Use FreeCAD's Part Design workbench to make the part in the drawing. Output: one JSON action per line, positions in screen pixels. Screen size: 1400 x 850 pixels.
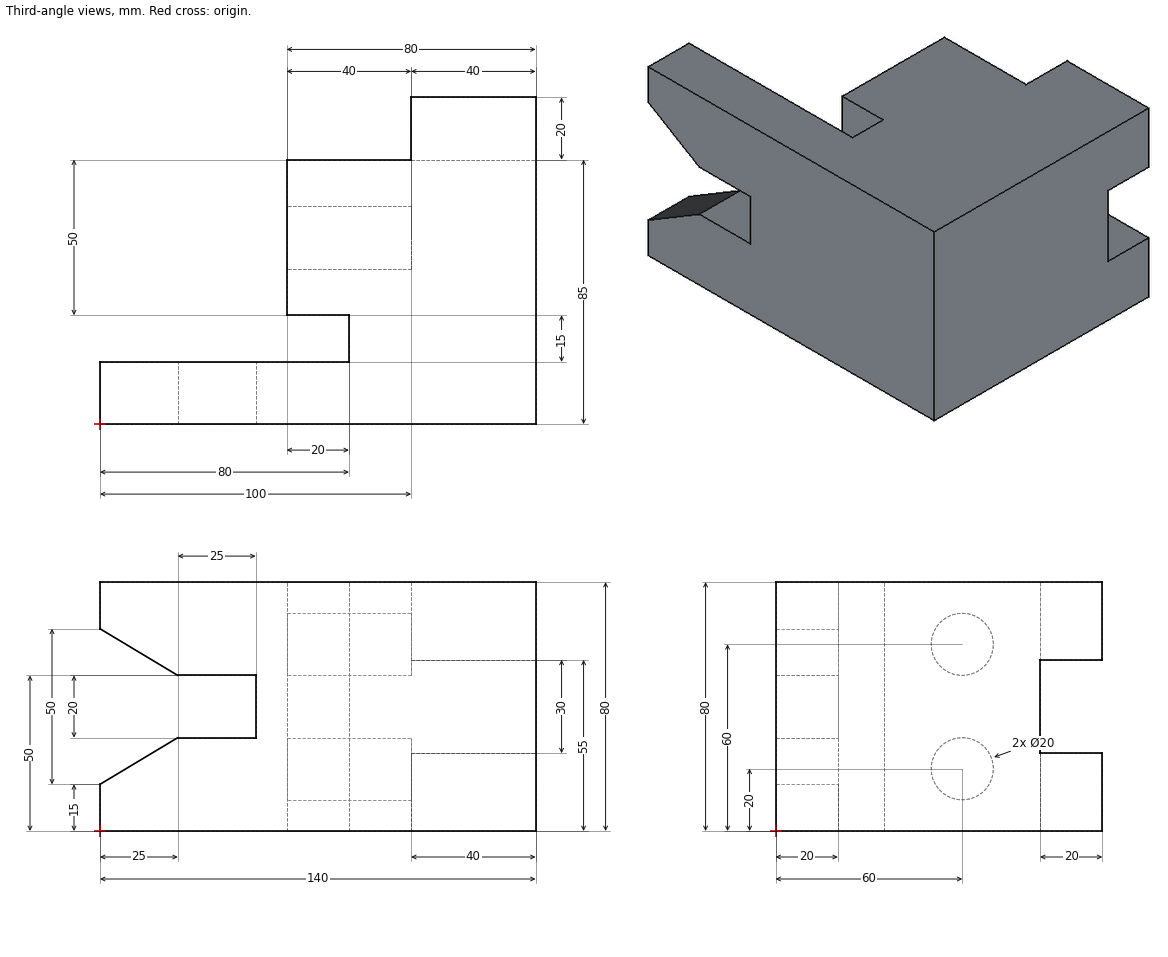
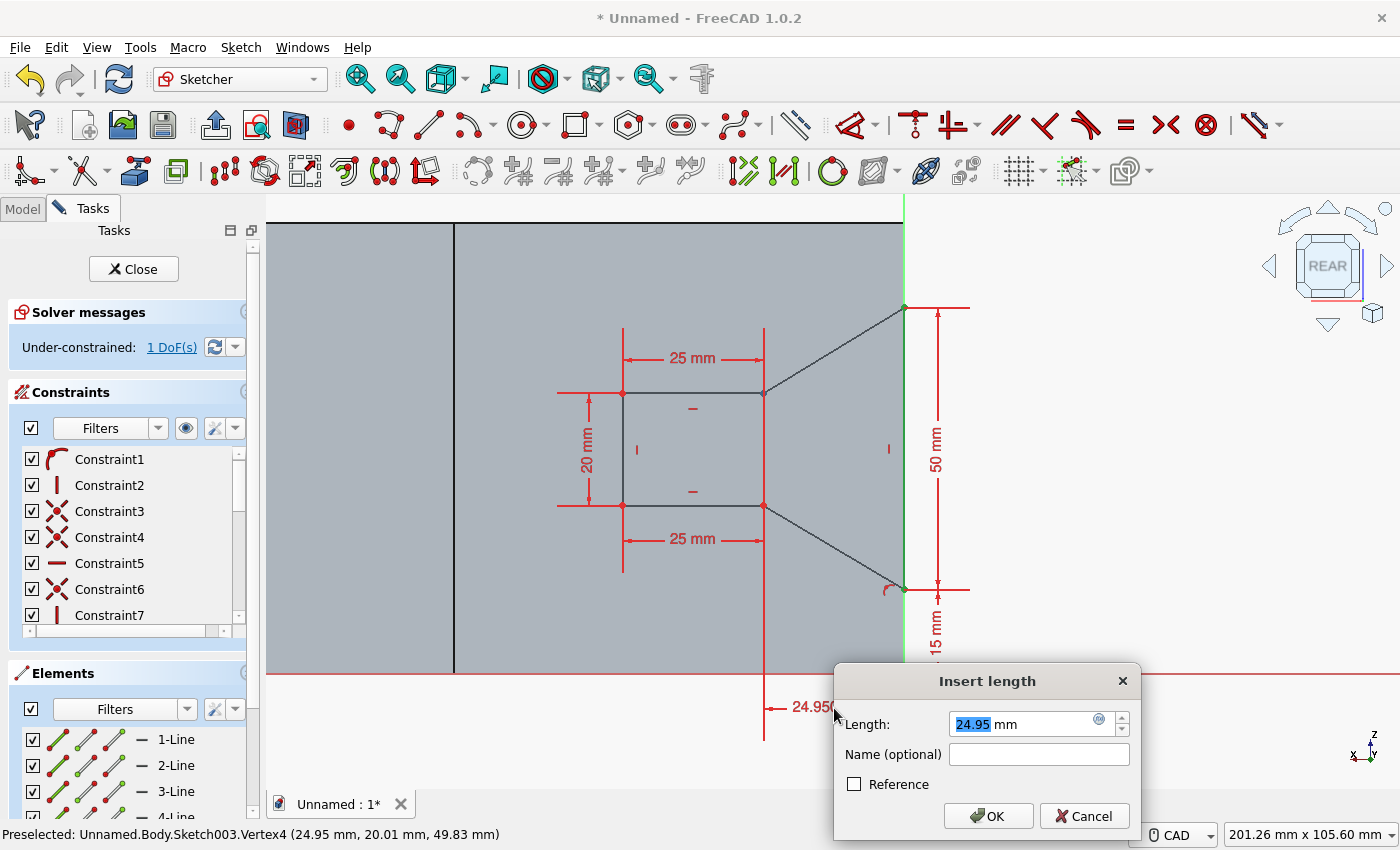
{"action": "type", "text": "25"}
{"action": "key", "text": "Return"}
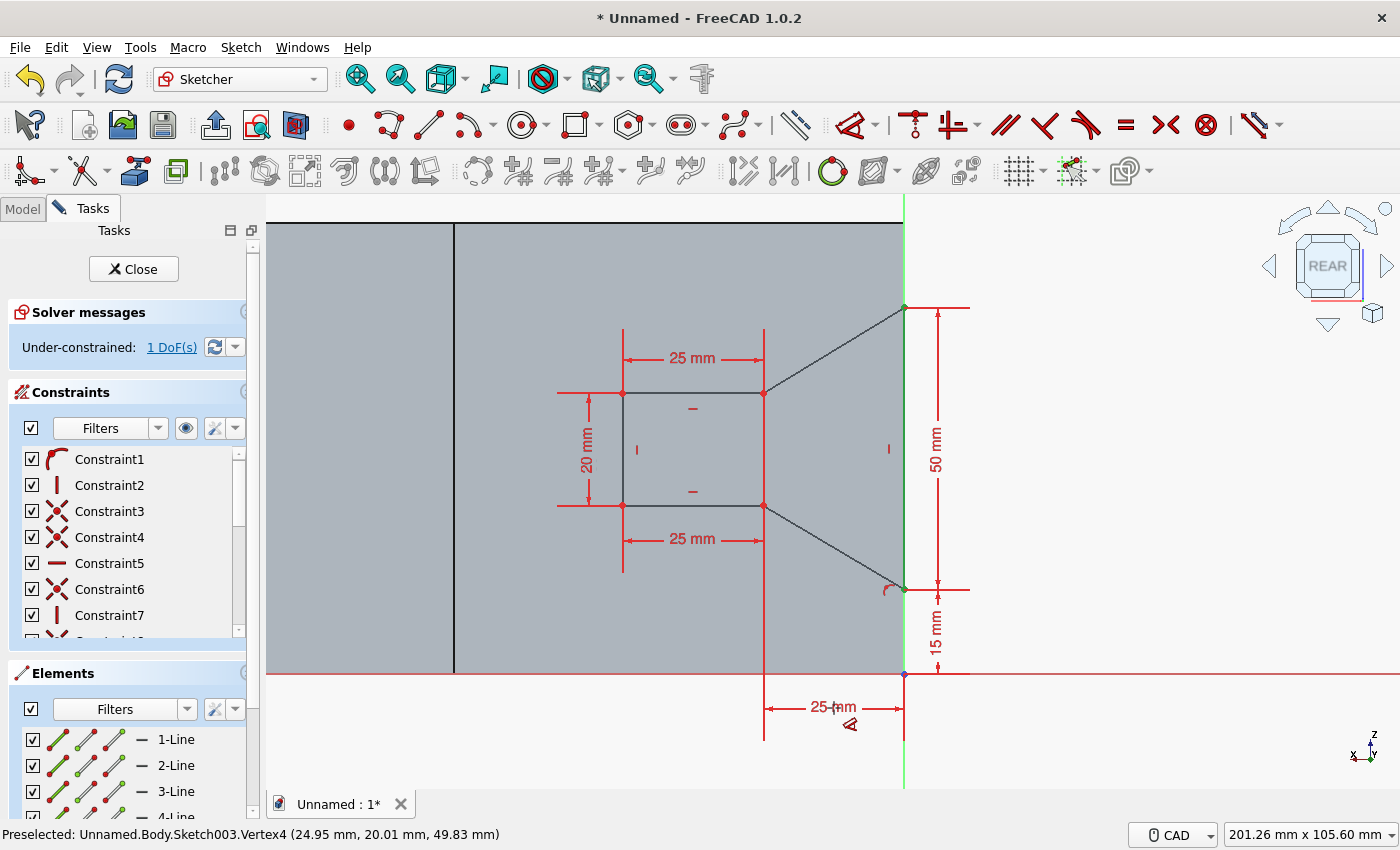
{"action": "left_click", "coordinate": [764, 393]}
{"action": "left_click", "coordinate": [938, 534]}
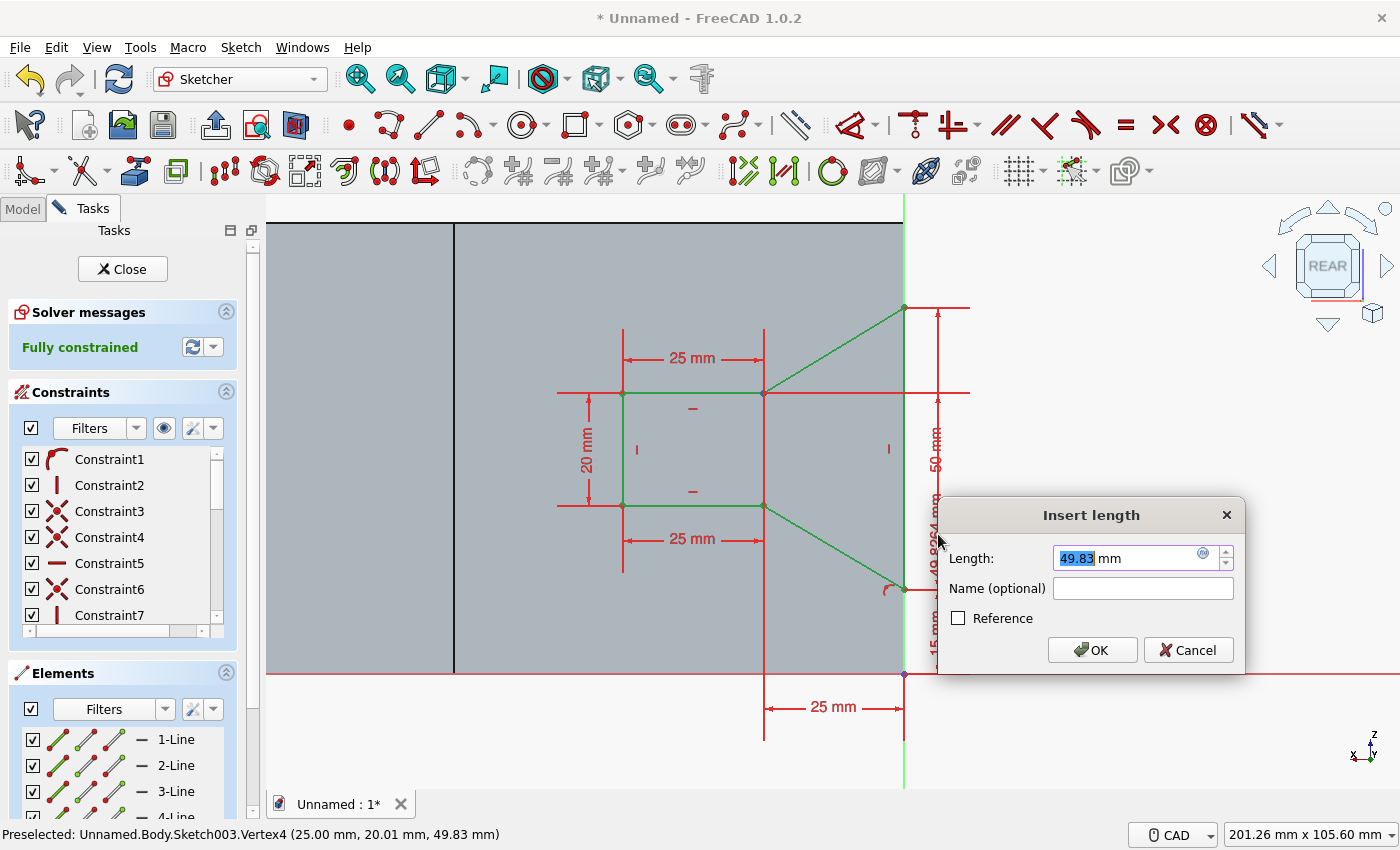
{"action": "type", "text": "50"}
{"action": "key", "text": "Return"}
{"action": "key", "text": "Escape"}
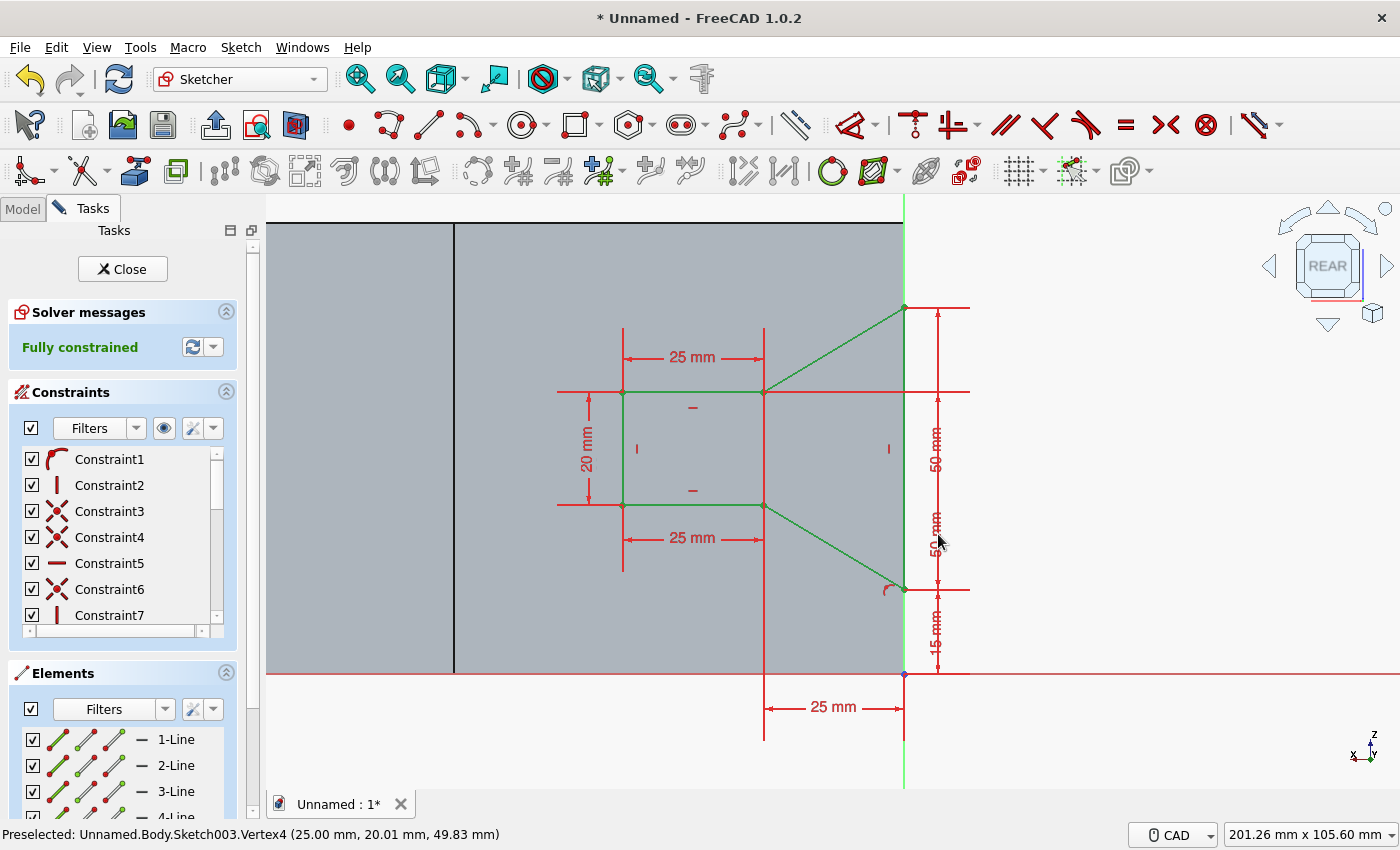
{"action": "left_click", "coordinate": [123, 269]}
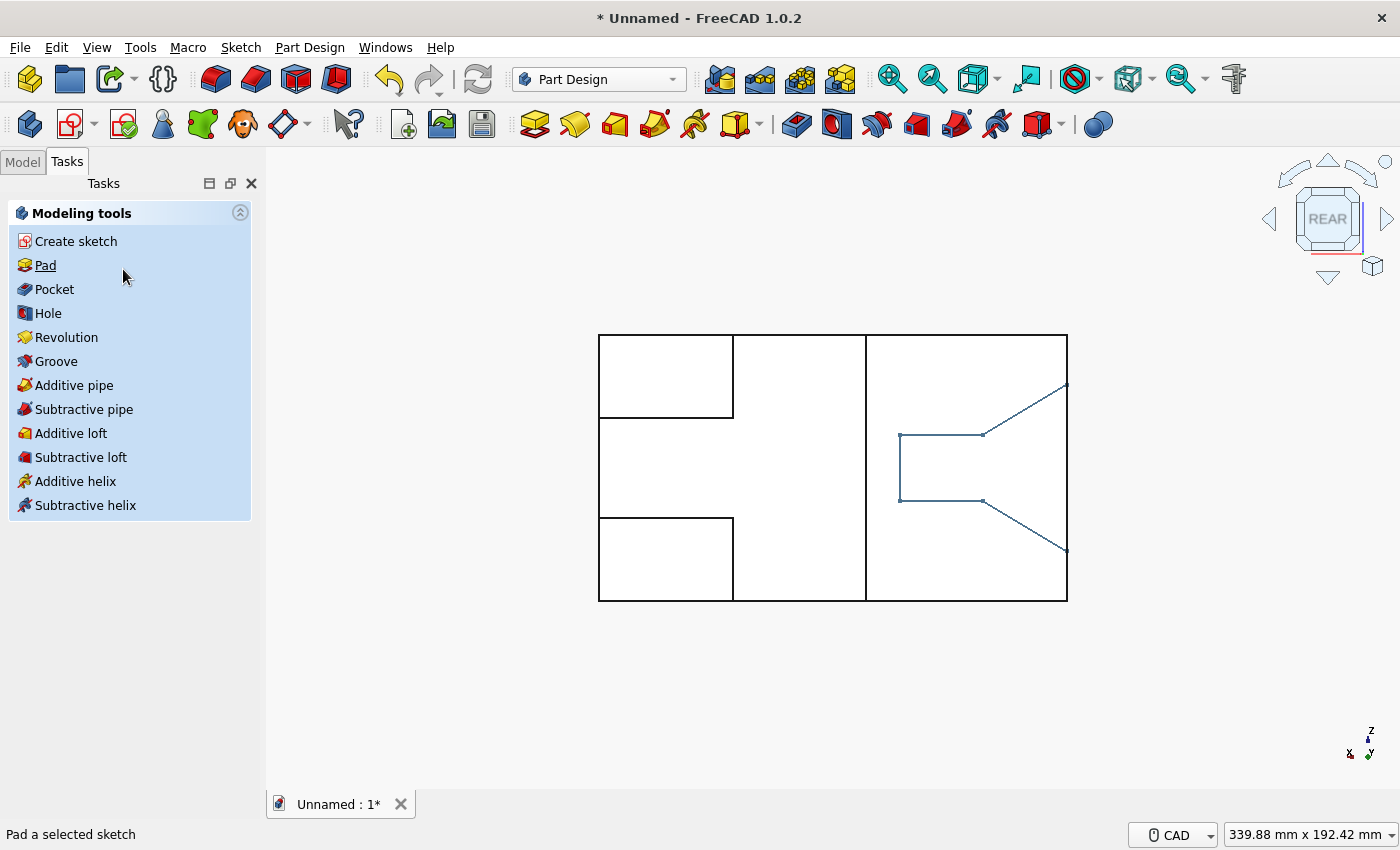
{"action": "left_click", "coordinate": [798, 124]}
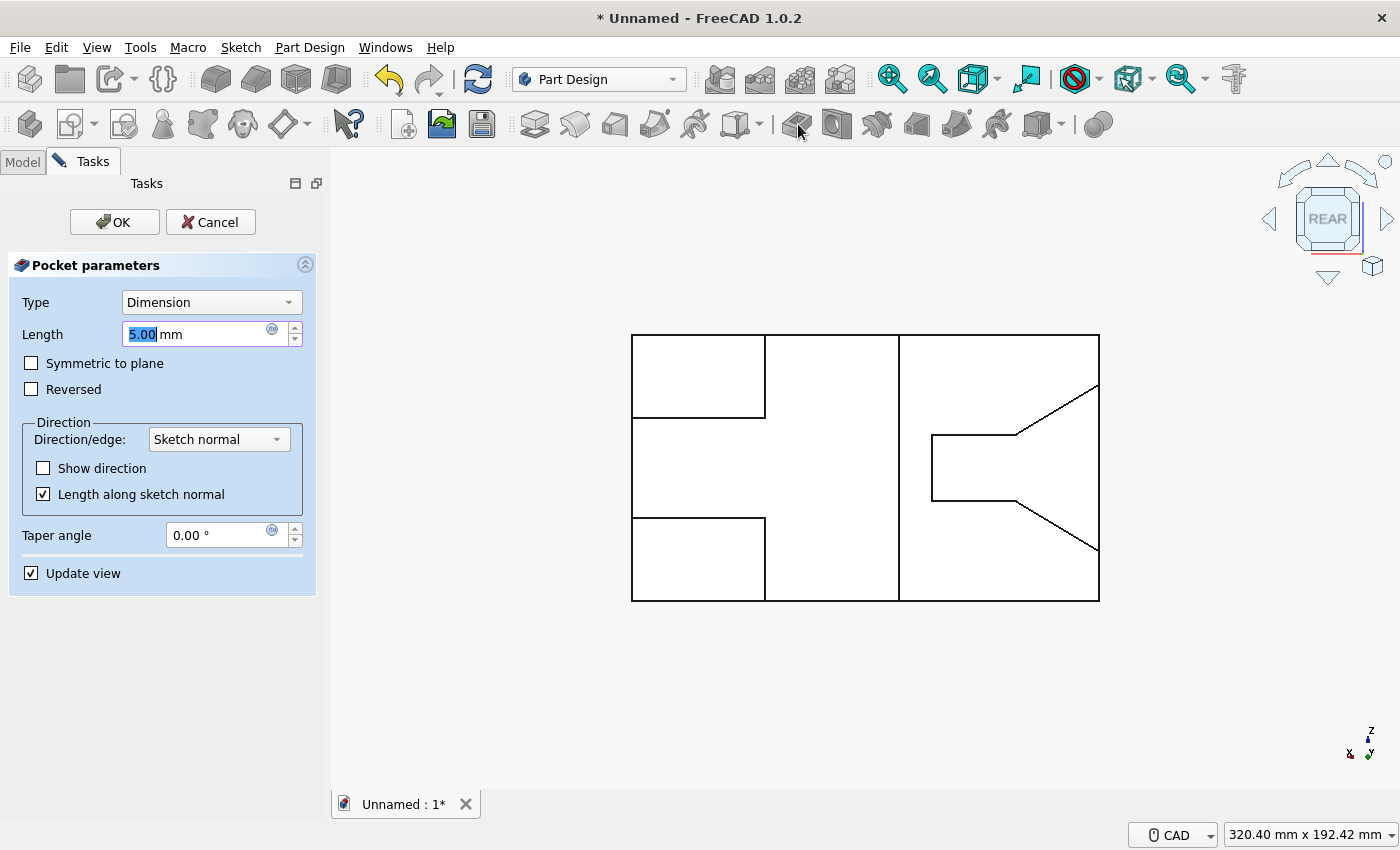
{"action": "left_click", "coordinate": [212, 302]}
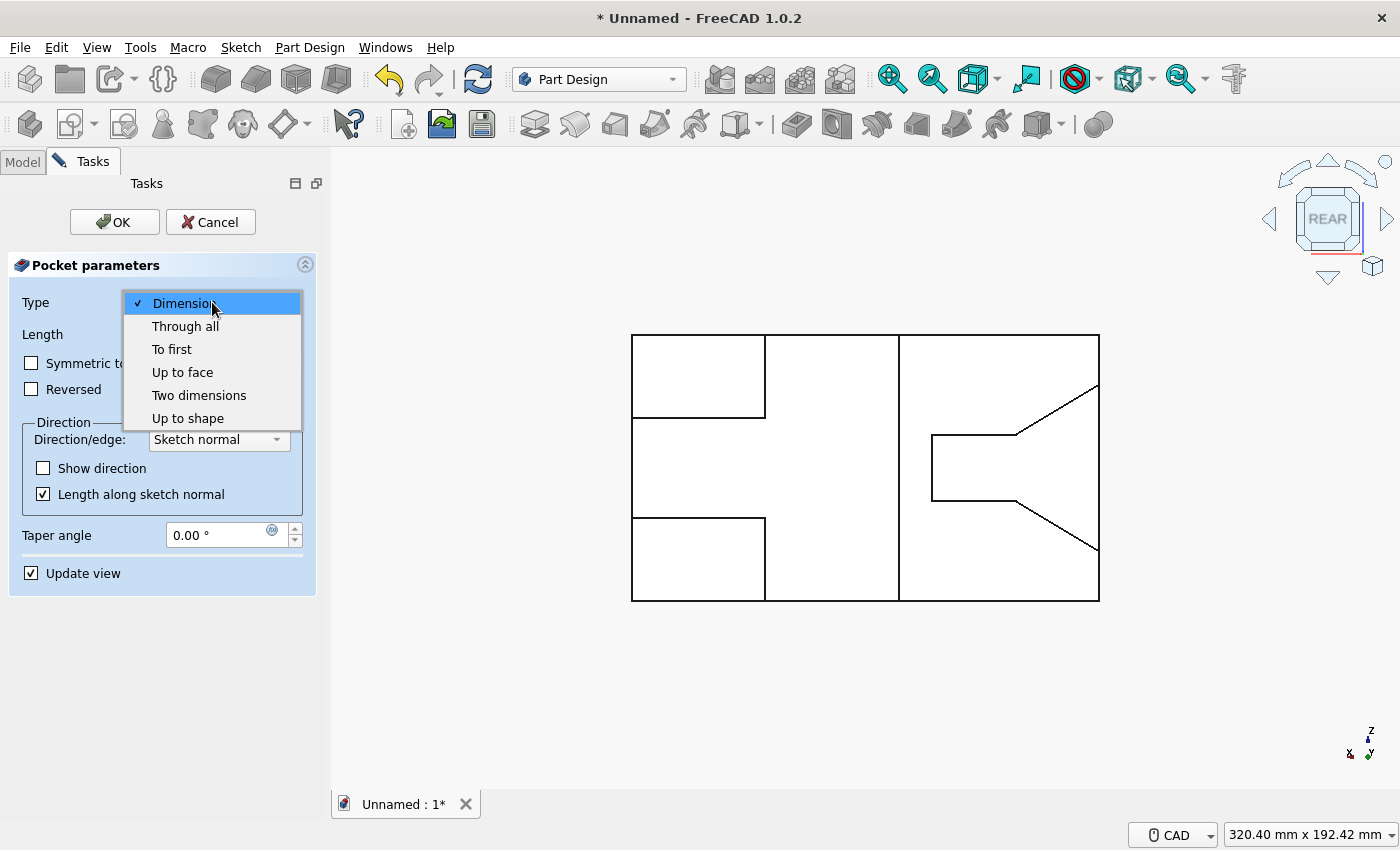
{"action": "left_click", "coordinate": [212, 396]}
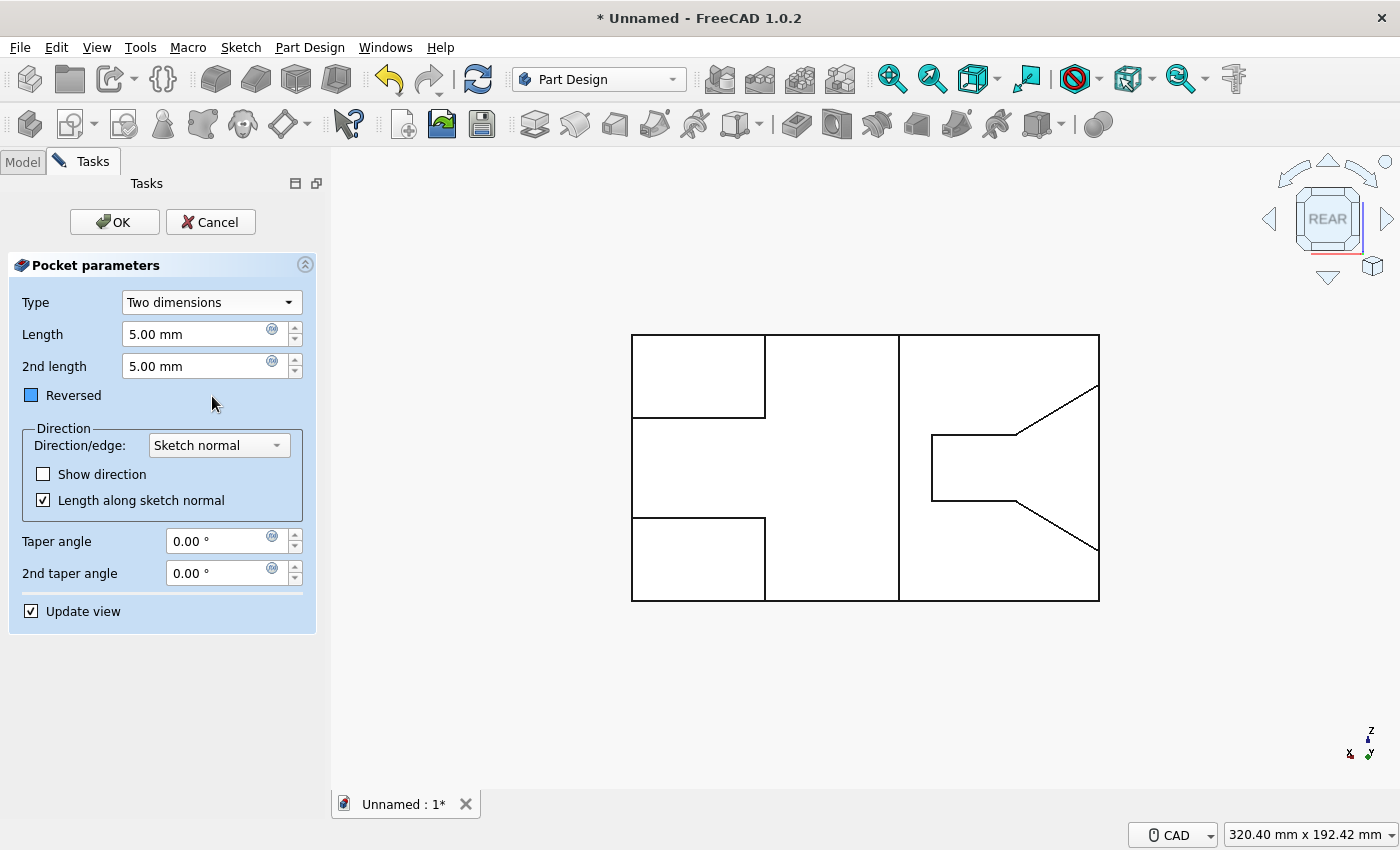
{"action": "triple_click", "coordinate": [204, 334]}